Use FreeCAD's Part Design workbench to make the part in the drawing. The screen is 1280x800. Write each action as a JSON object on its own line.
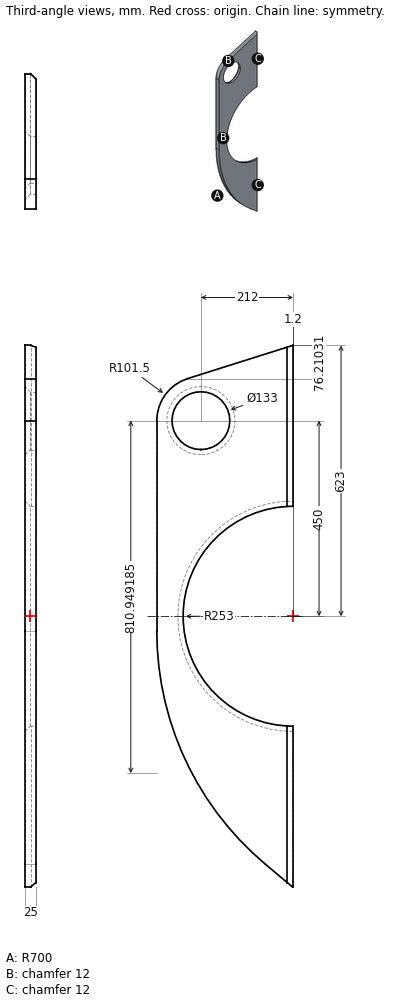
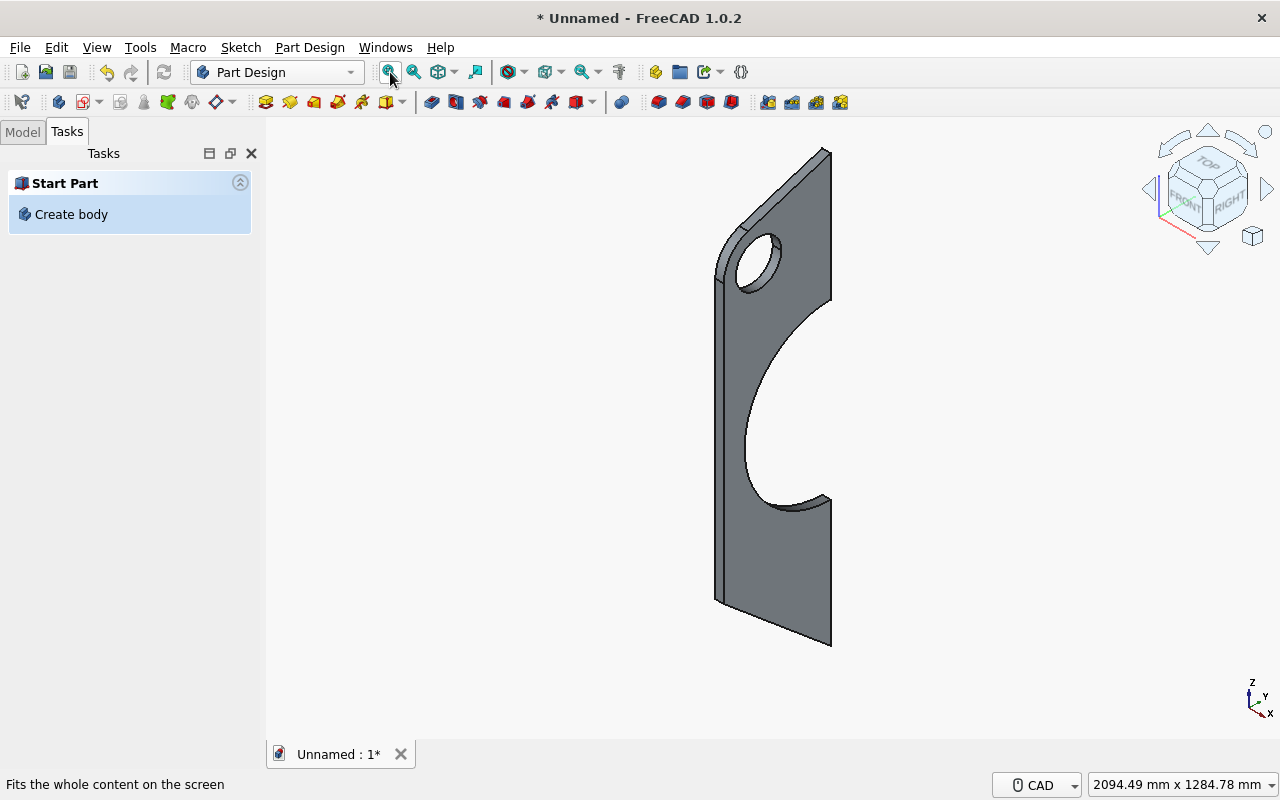
{"action": "scroll", "coordinate": [720, 601], "scroll_direction": "up", "scroll_amount": 6}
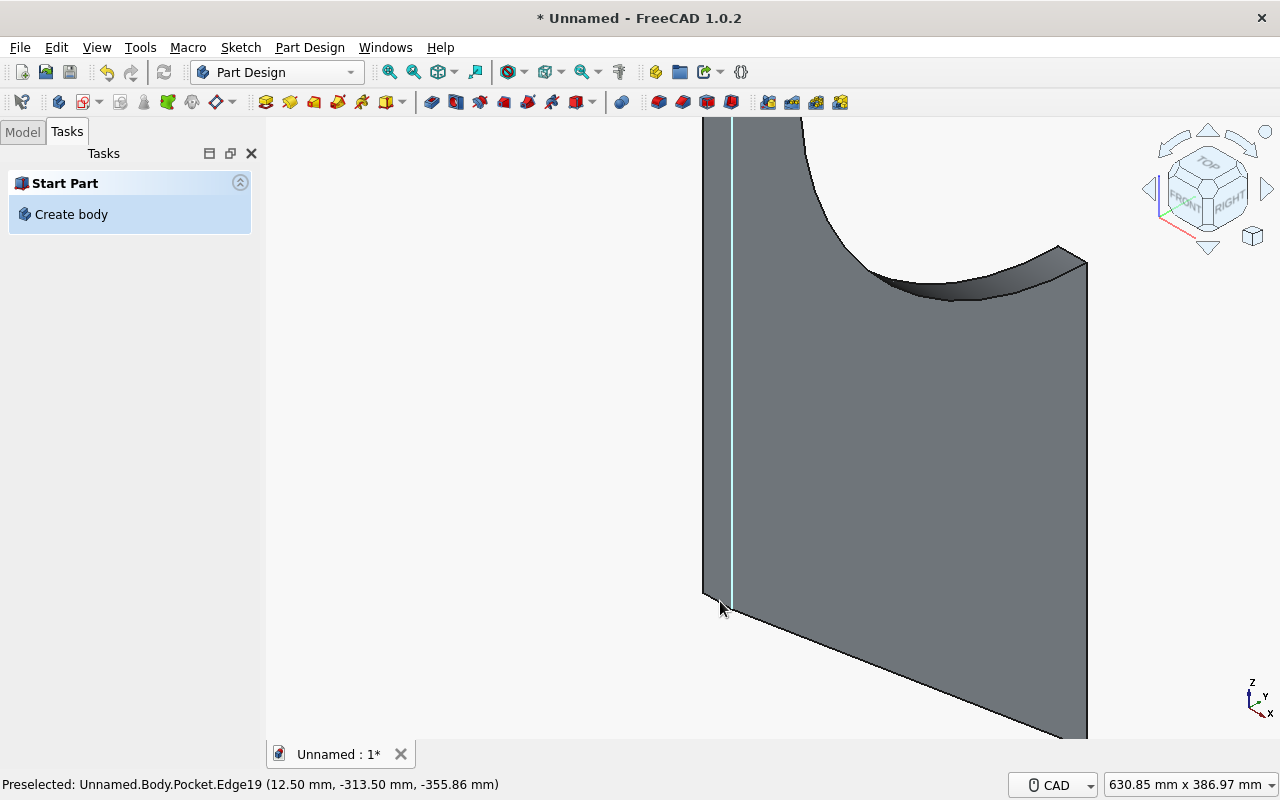
{"action": "left_click", "coordinate": [390, 72]}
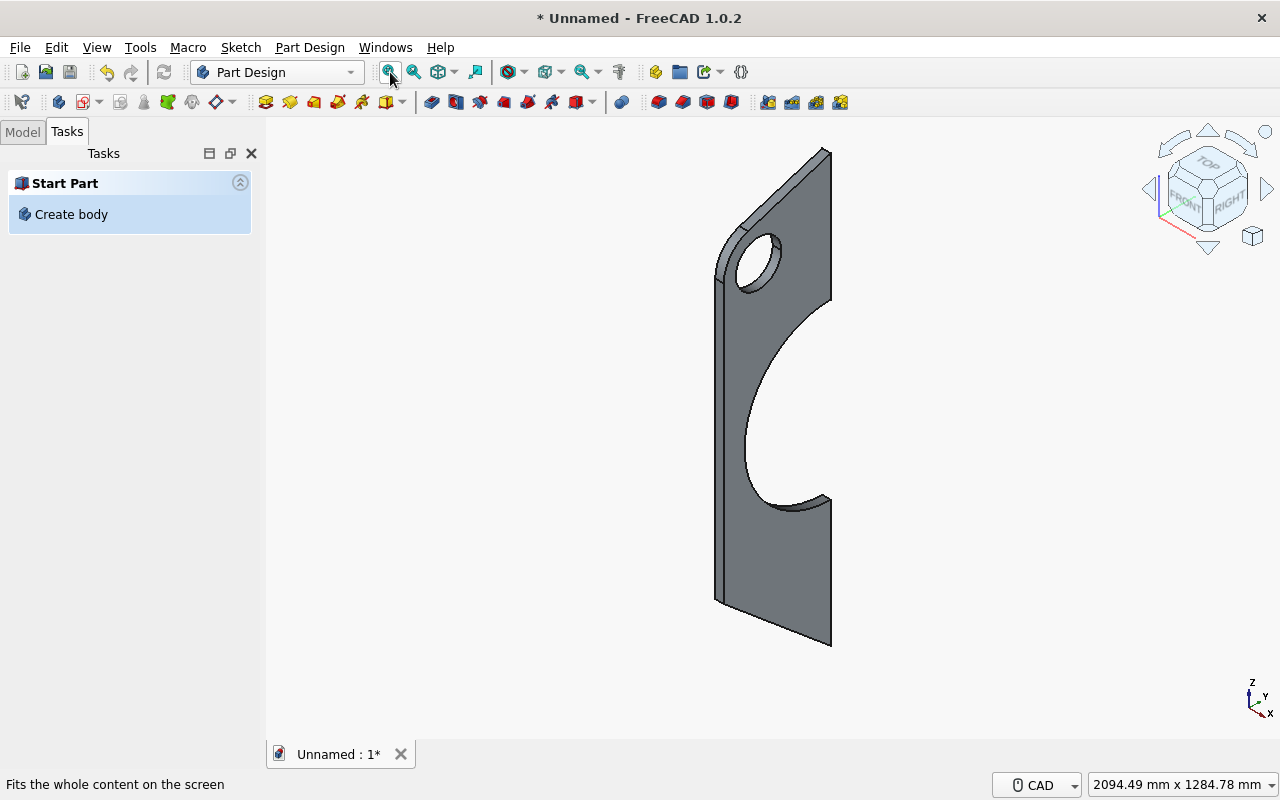
{"action": "key", "text": "2"}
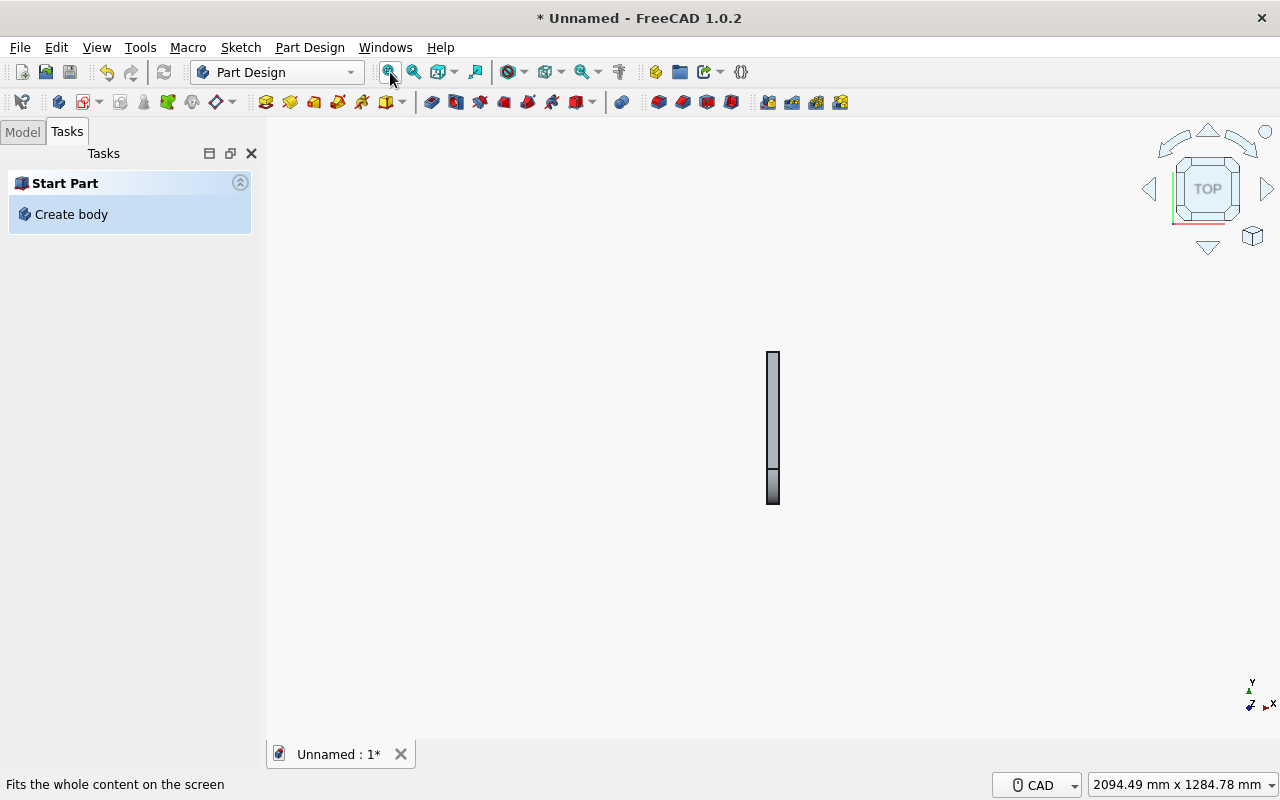
{"action": "left_click", "coordinate": [390, 72]}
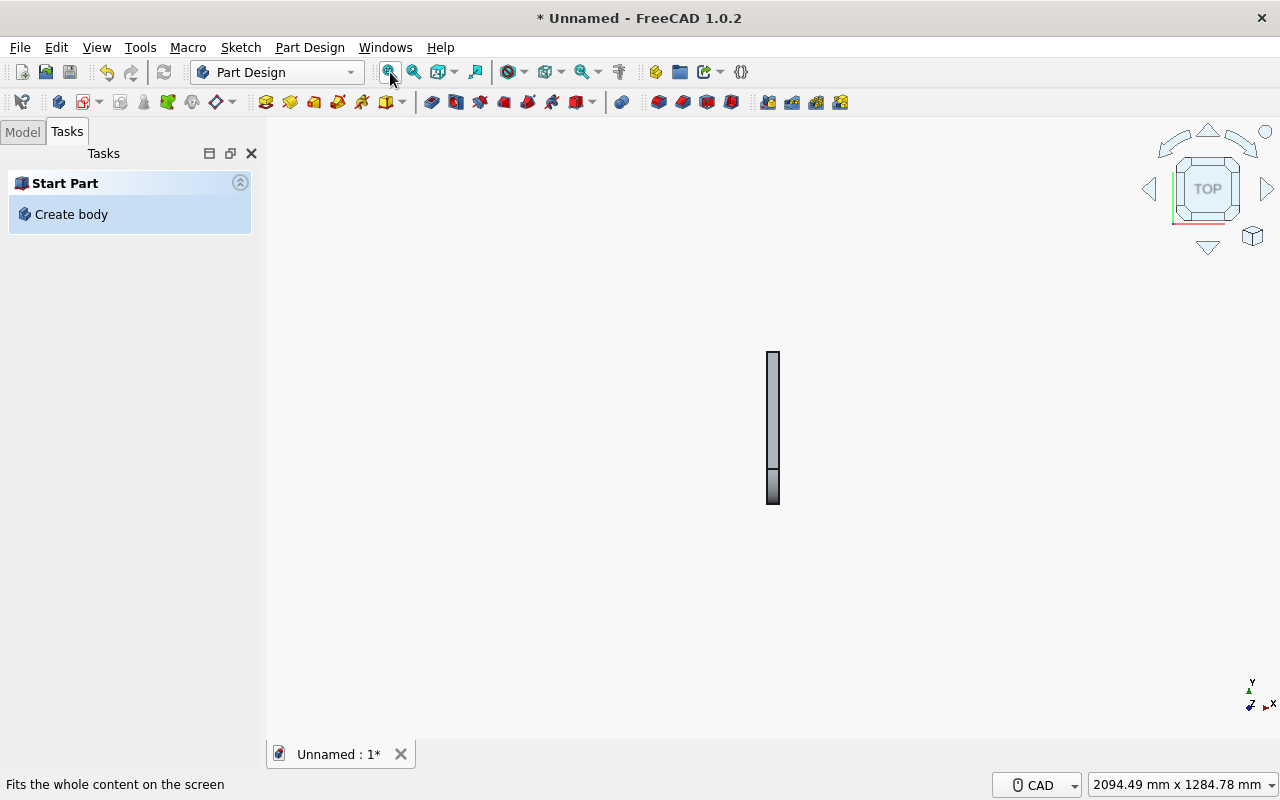
{"action": "scroll", "coordinate": [773, 503], "scroll_direction": "up", "scroll_amount": 6}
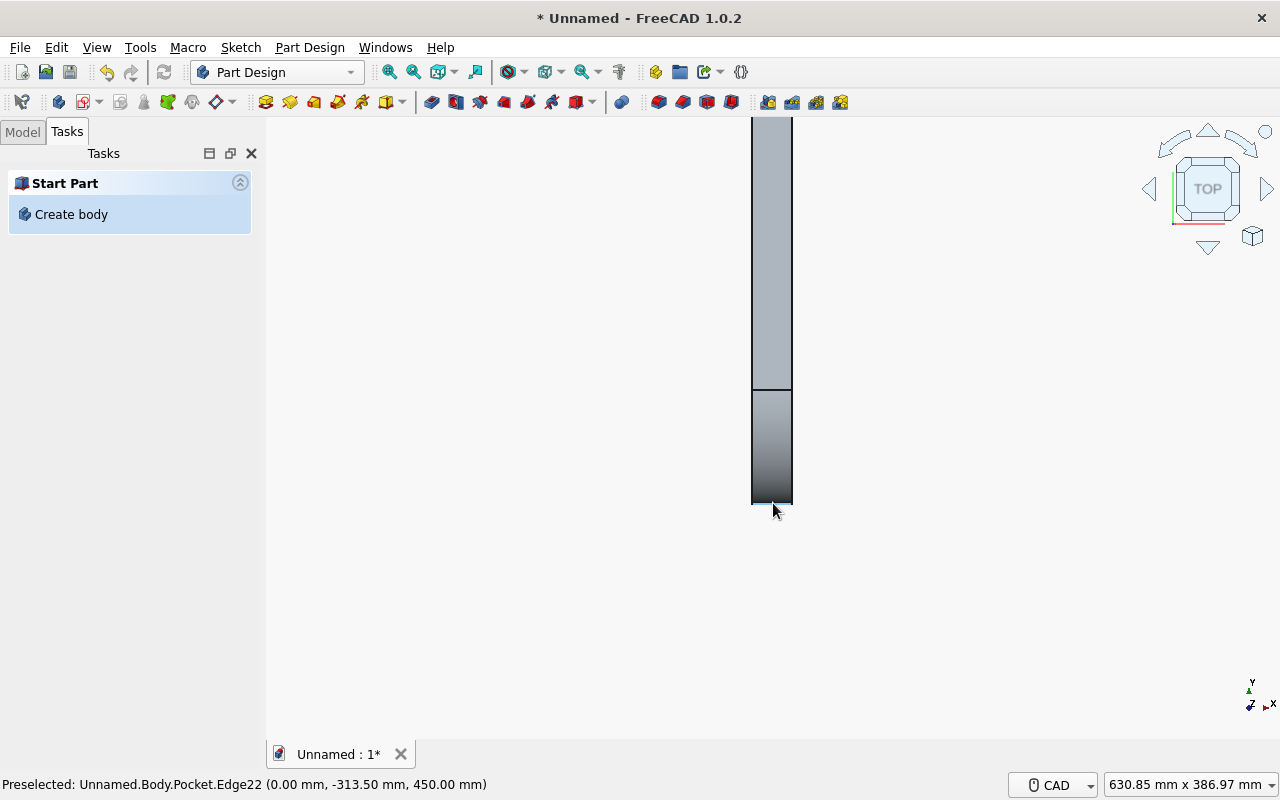
{"action": "left_click", "coordinate": [390, 72]}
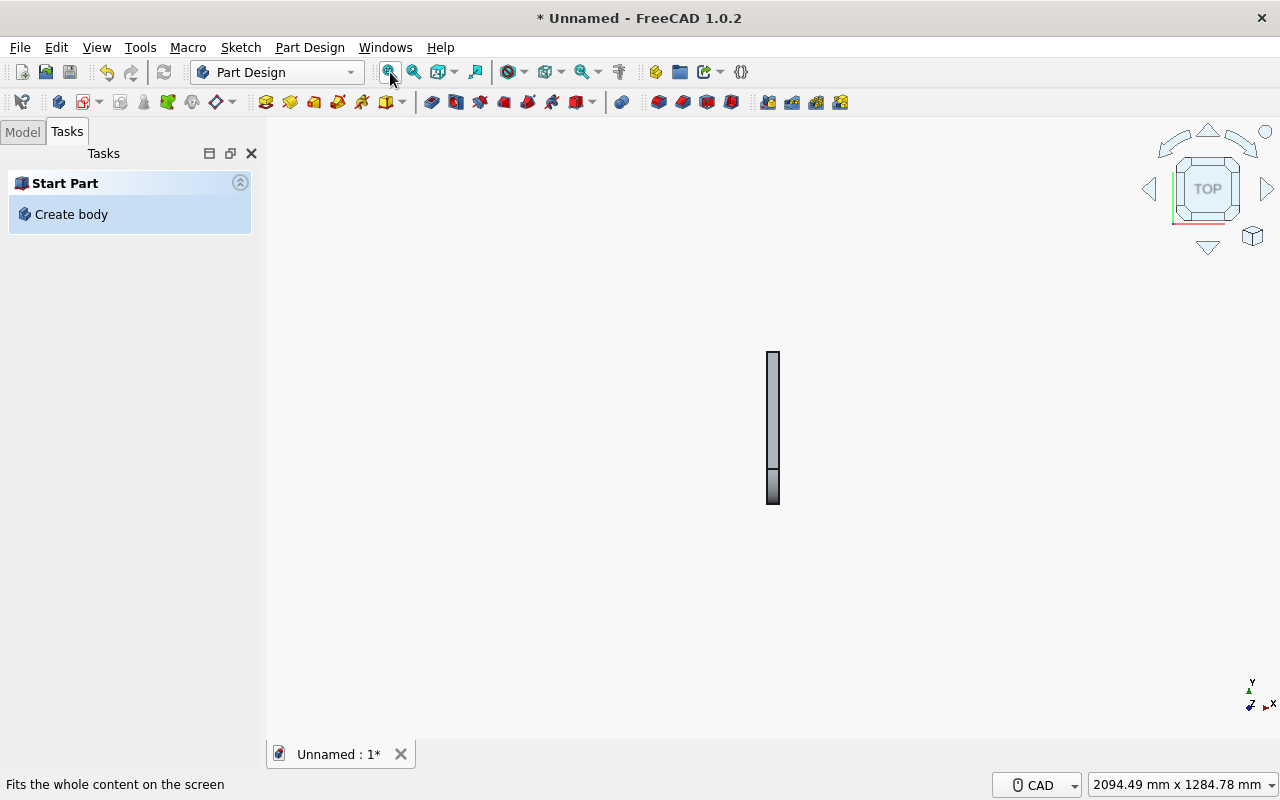
{"action": "key", "text": "1"}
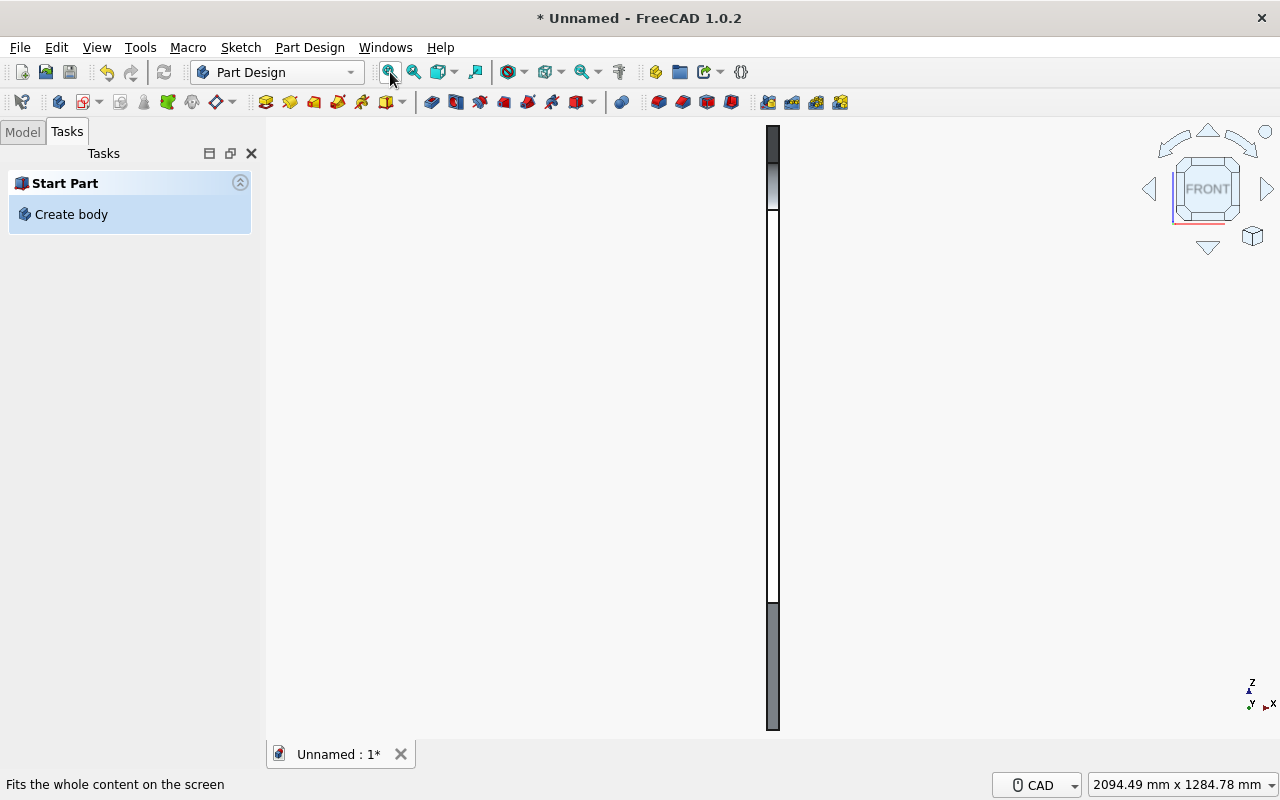
{"action": "left_click", "coordinate": [773, 602]}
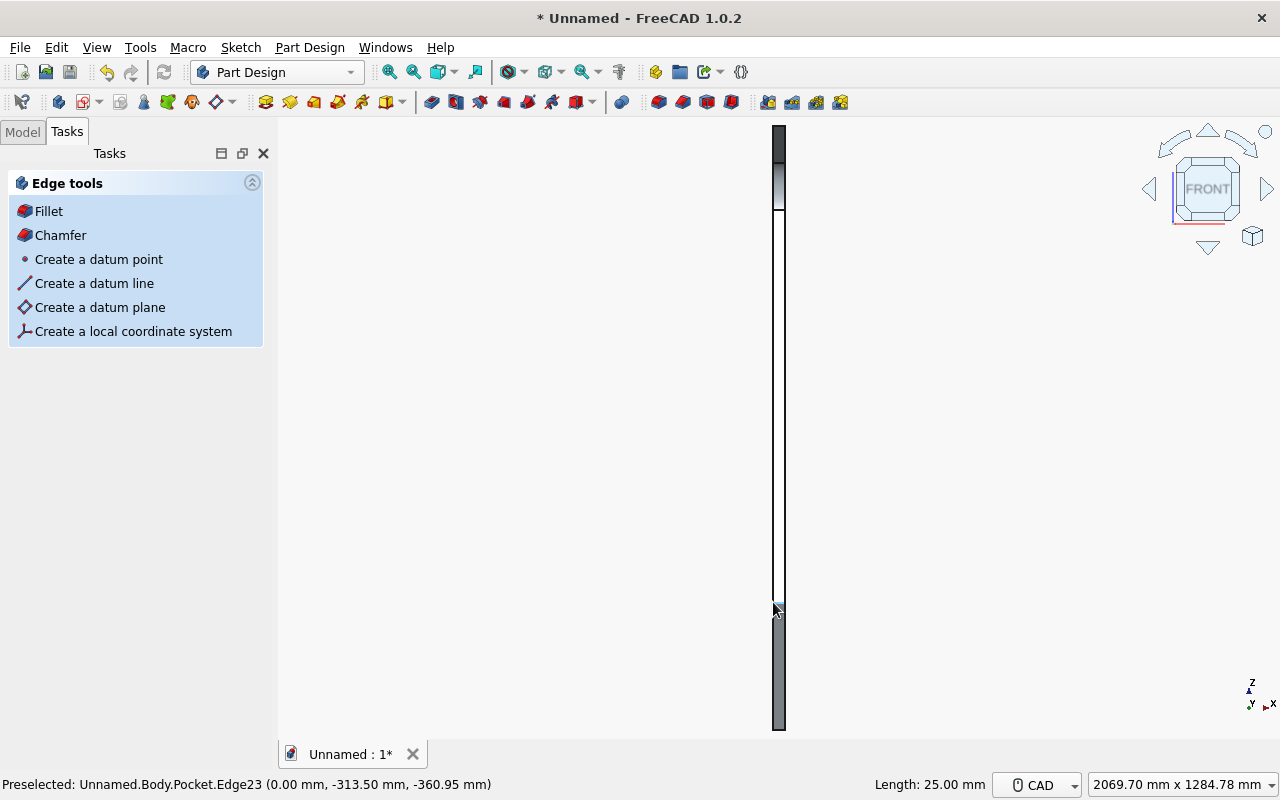
{"action": "left_click", "coordinate": [660, 102]}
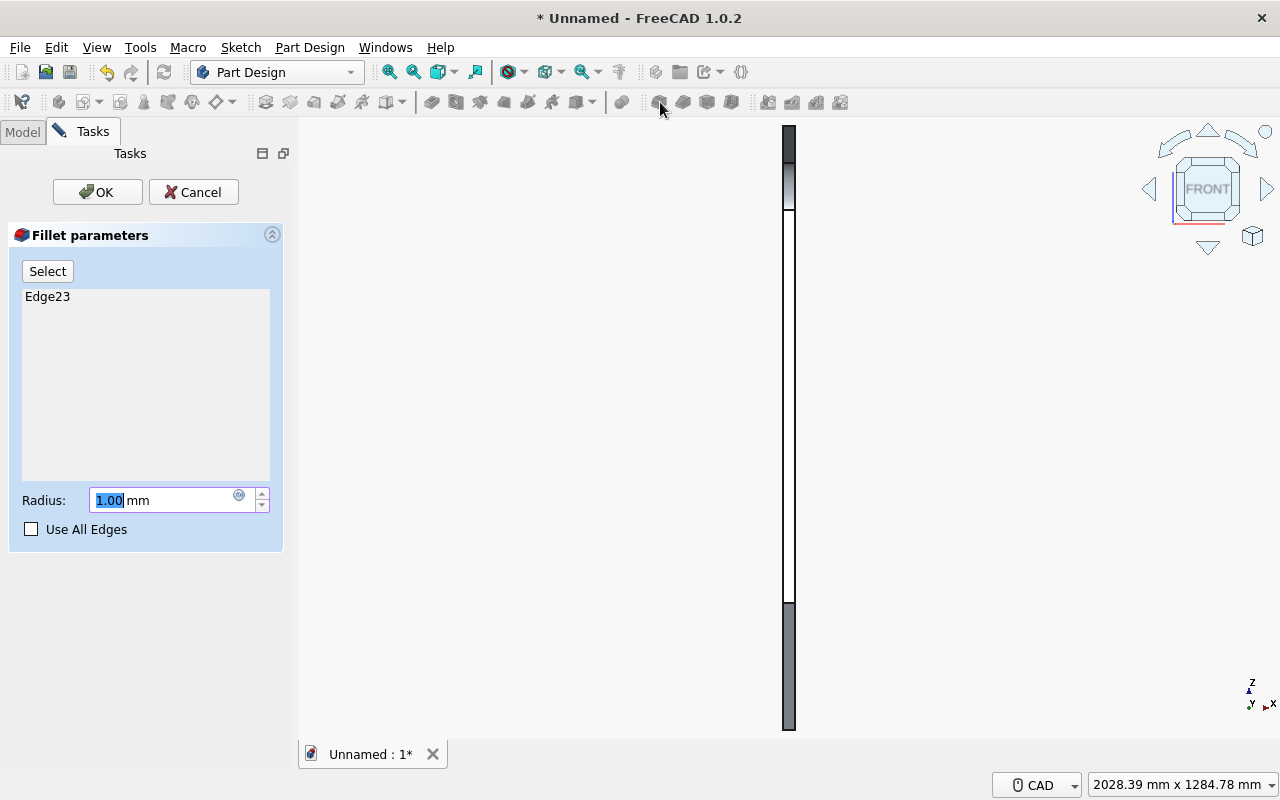
{"action": "type", "text": "700"}
{"action": "key", "text": "Tab"}